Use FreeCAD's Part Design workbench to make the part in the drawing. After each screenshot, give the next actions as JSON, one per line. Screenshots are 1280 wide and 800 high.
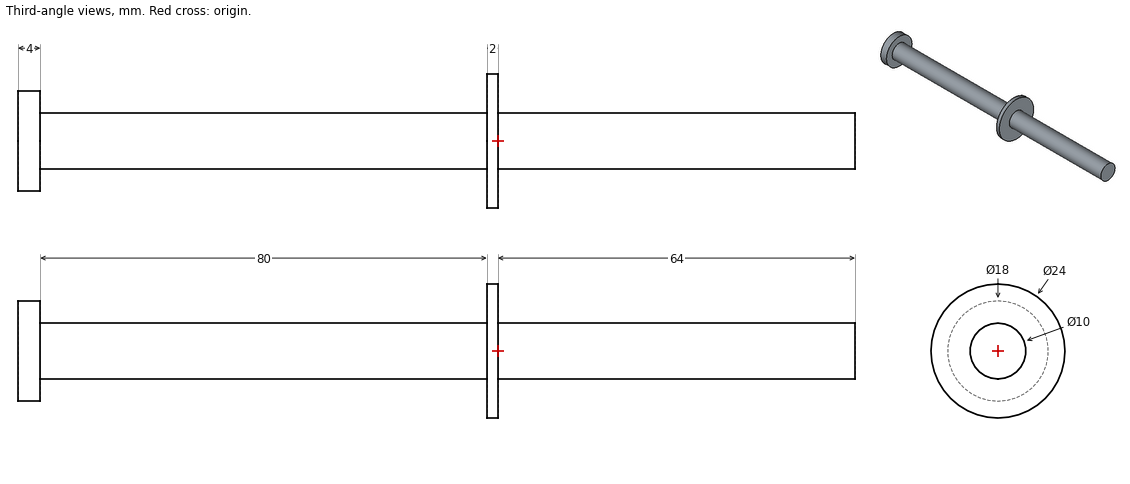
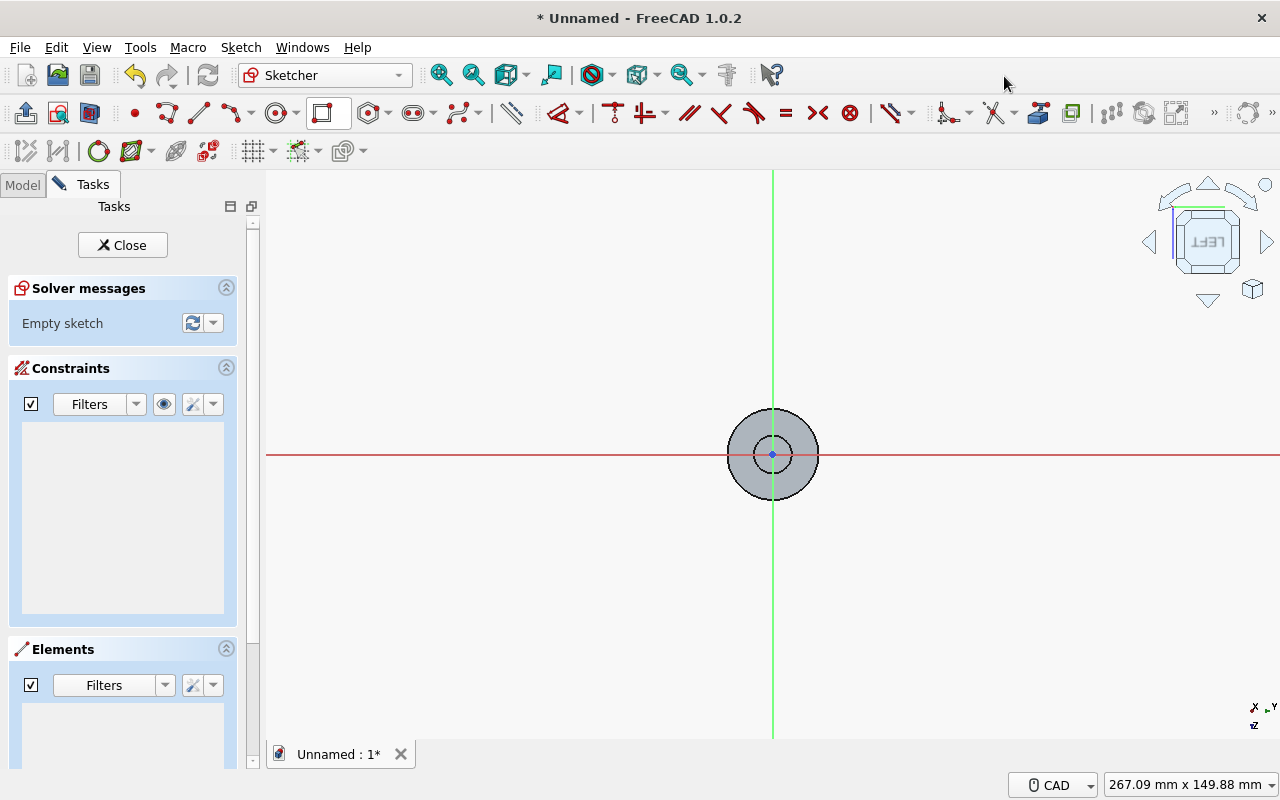
{"action": "scroll", "coordinate": [790, 454], "scroll_direction": "up", "scroll_amount": 8}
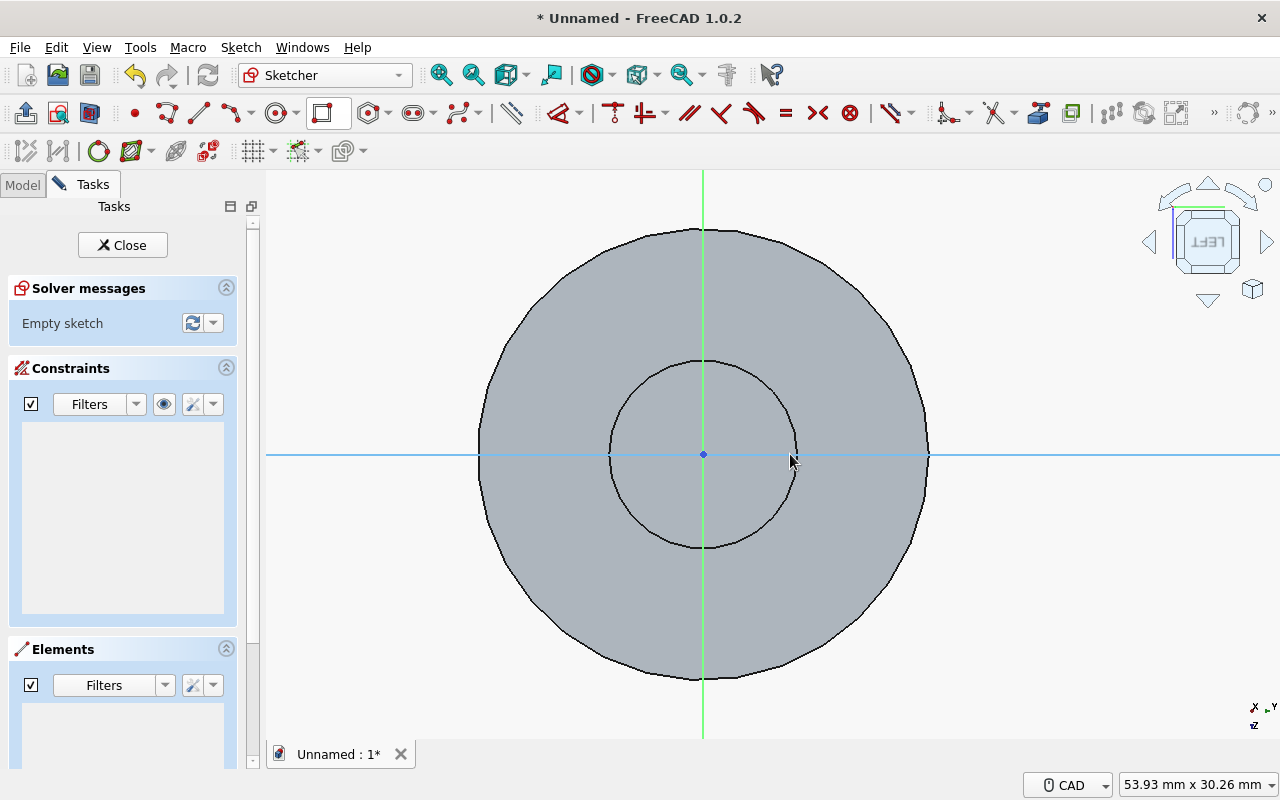
{"action": "left_click", "coordinate": [276, 114]}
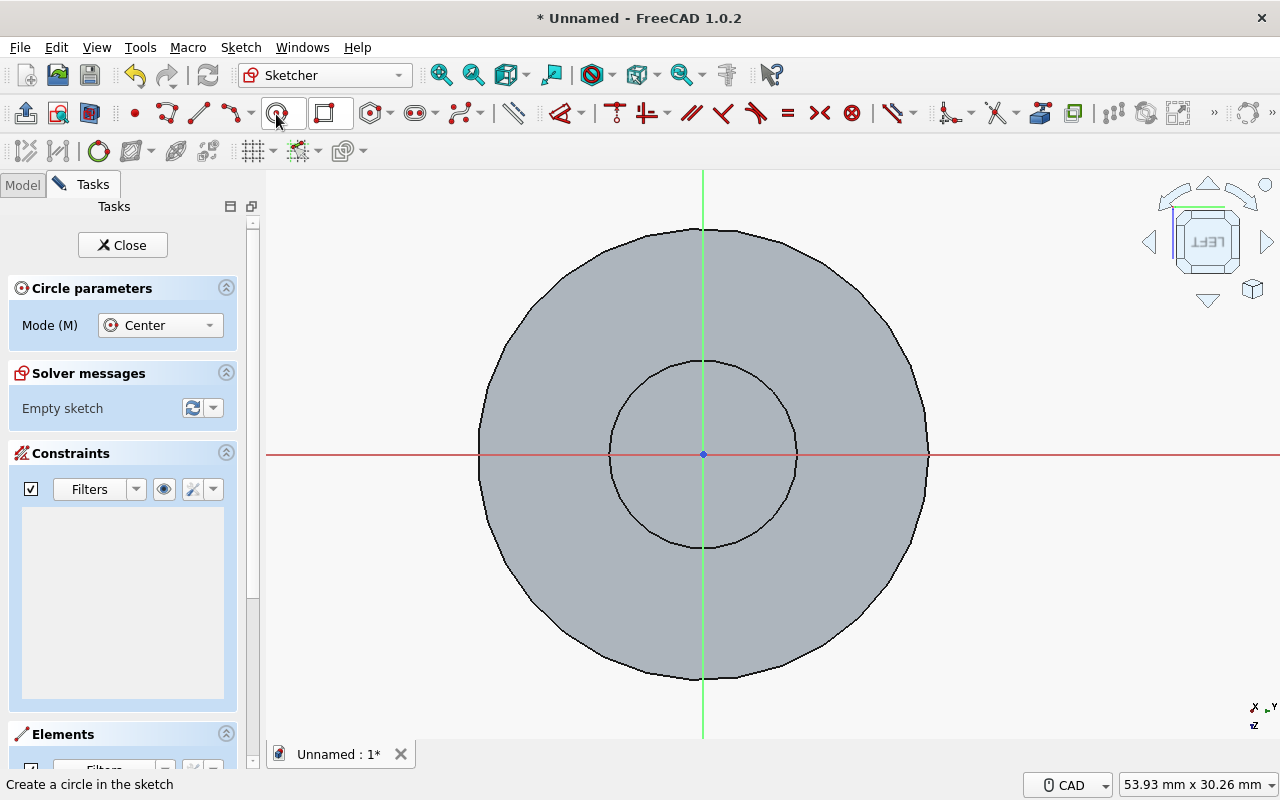
{"action": "left_click", "coordinate": [703, 454]}
{"action": "mouse_move", "coordinate": [823, 335]}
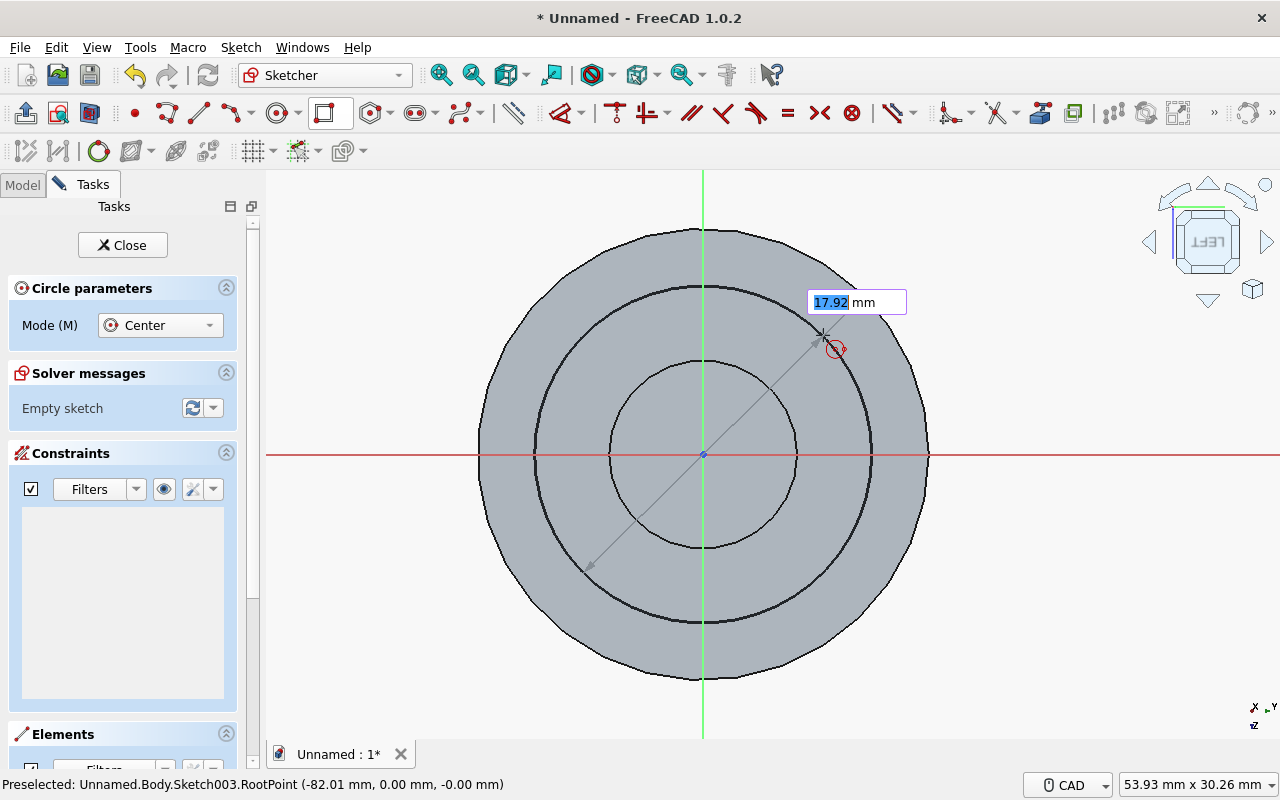
{"action": "type", "text": "18"}
{"action": "key", "text": "Return"}
{"action": "key", "text": "Escape"}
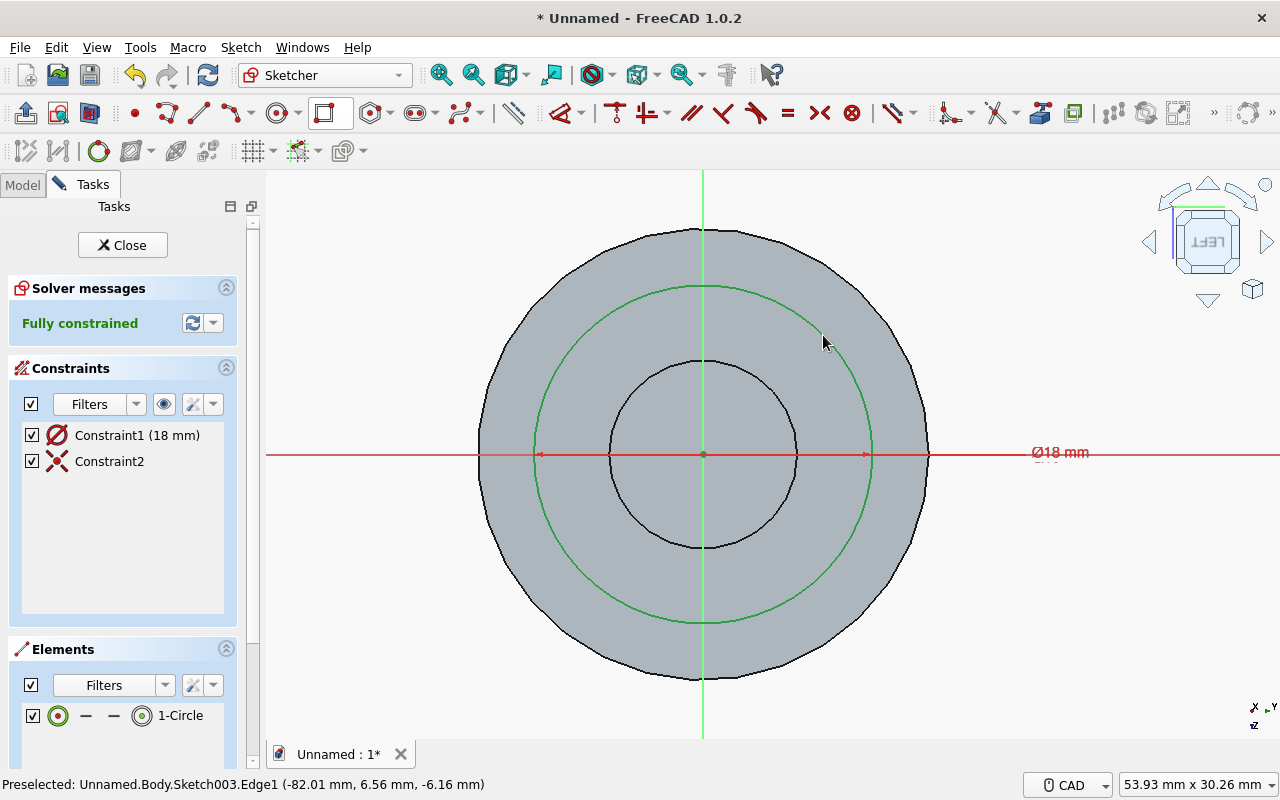
{"action": "left_click", "coordinate": [123, 245]}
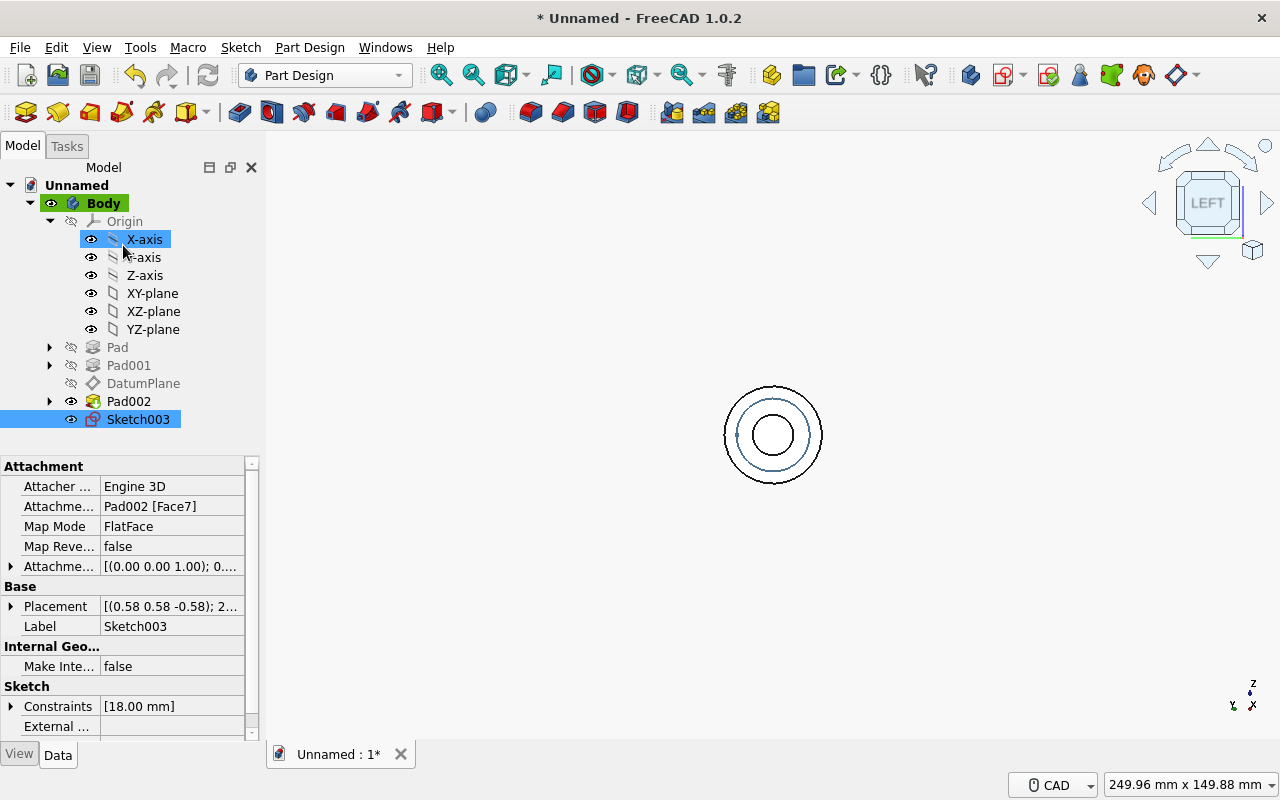
{"action": "left_click", "coordinate": [26, 112]}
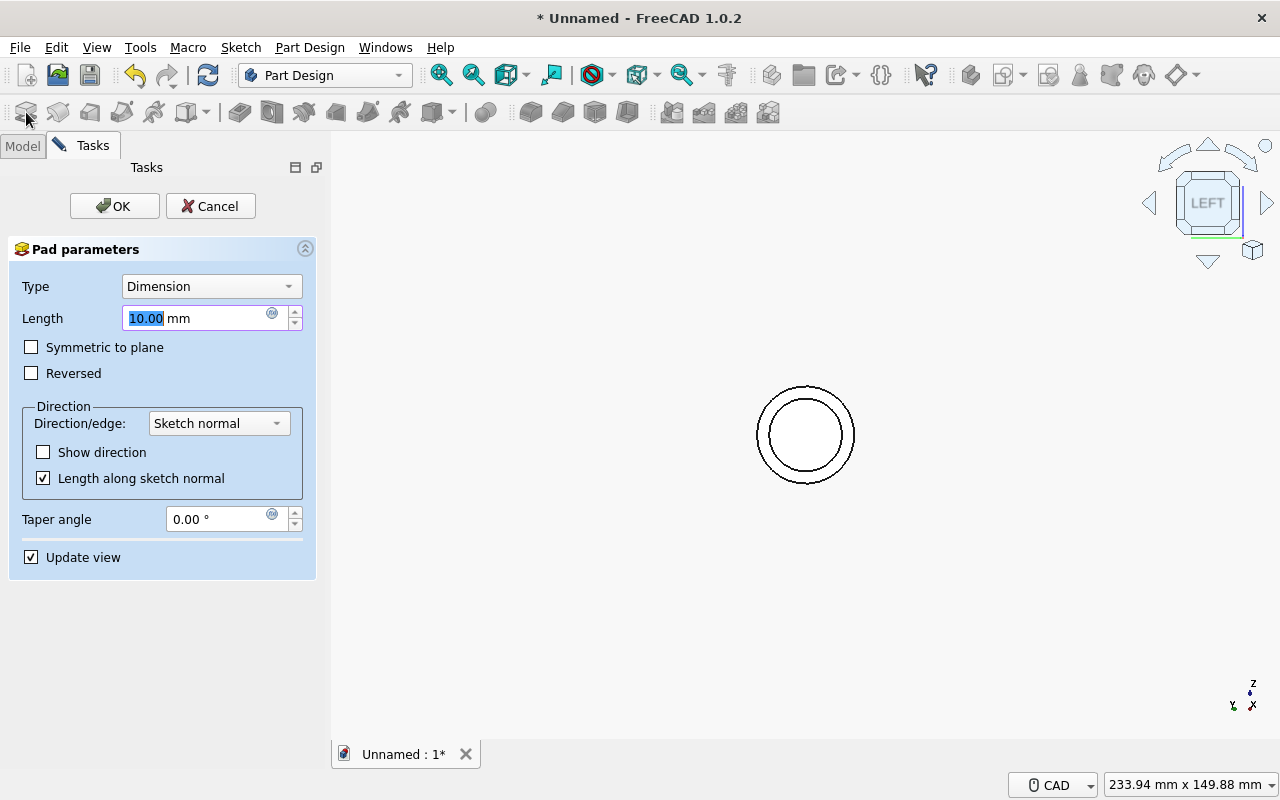
{"action": "type", "text": "4"}
{"action": "key", "text": "Tab"}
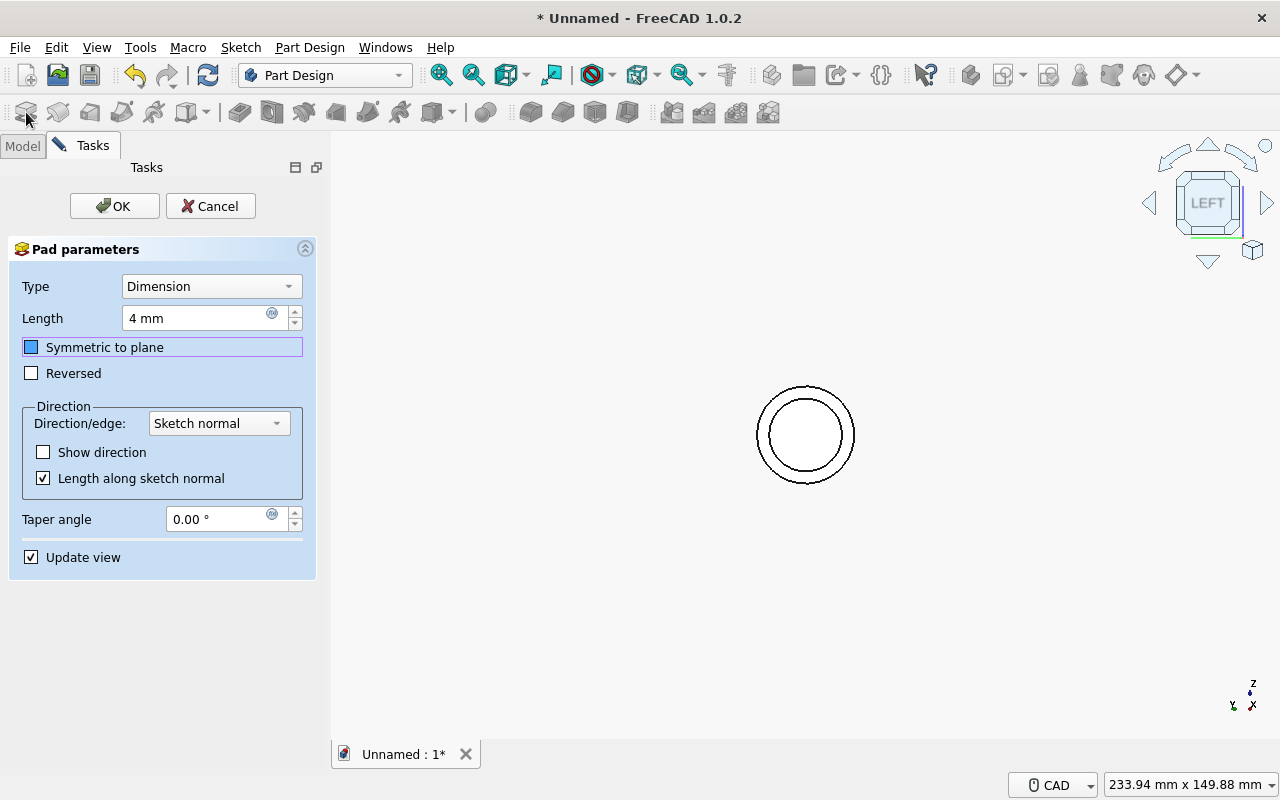
{"action": "left_click", "coordinate": [115, 206]}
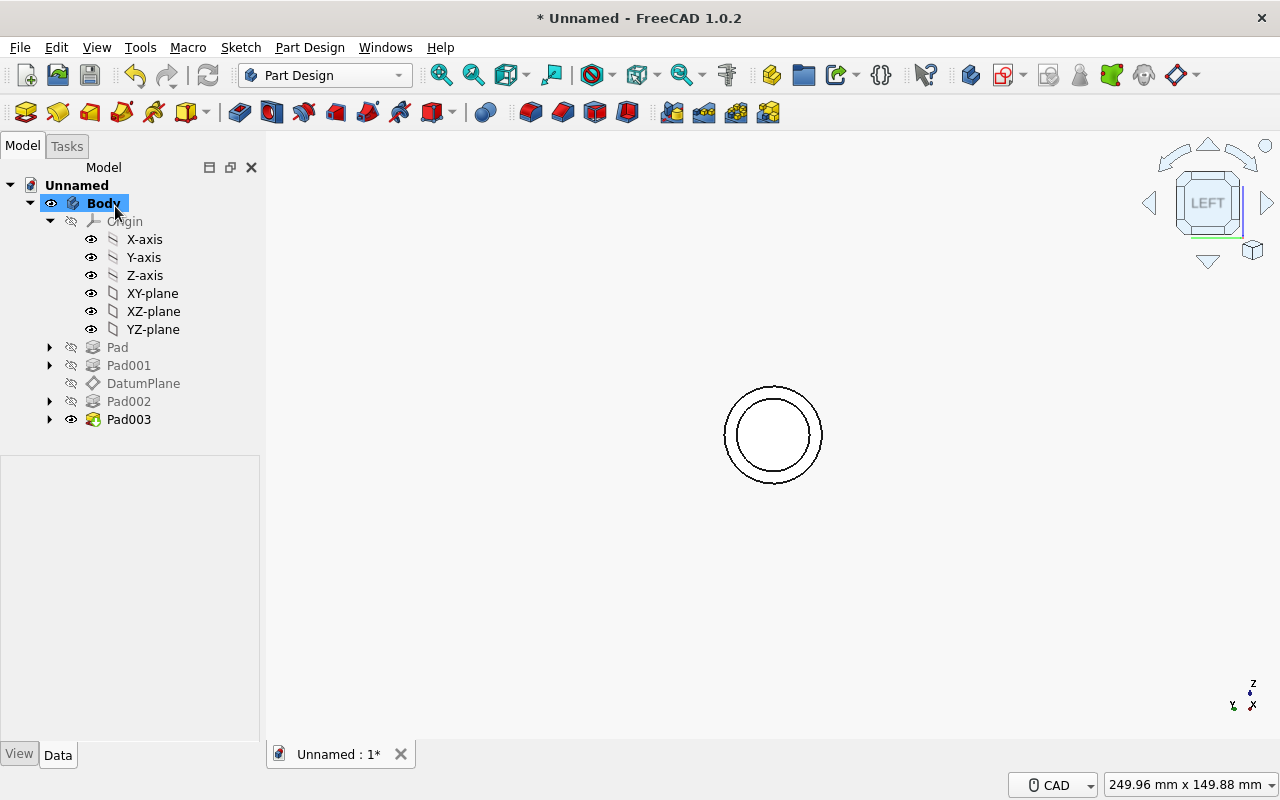
{"action": "key", "text": "0"}